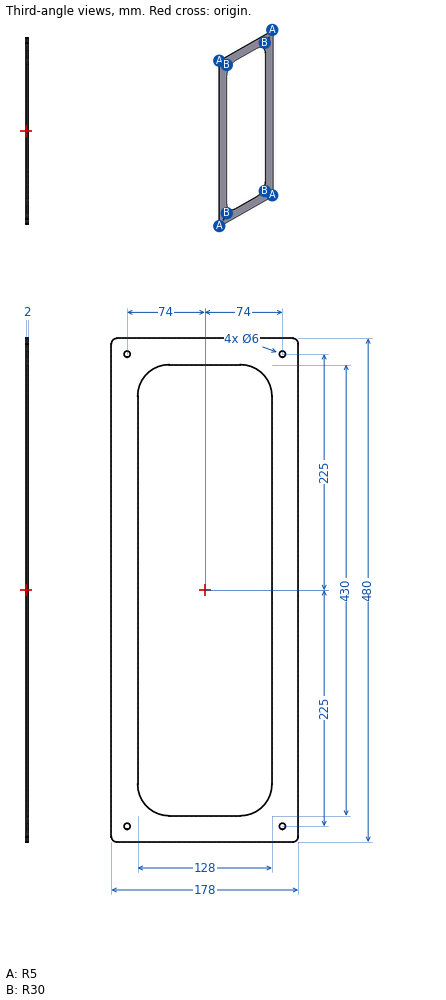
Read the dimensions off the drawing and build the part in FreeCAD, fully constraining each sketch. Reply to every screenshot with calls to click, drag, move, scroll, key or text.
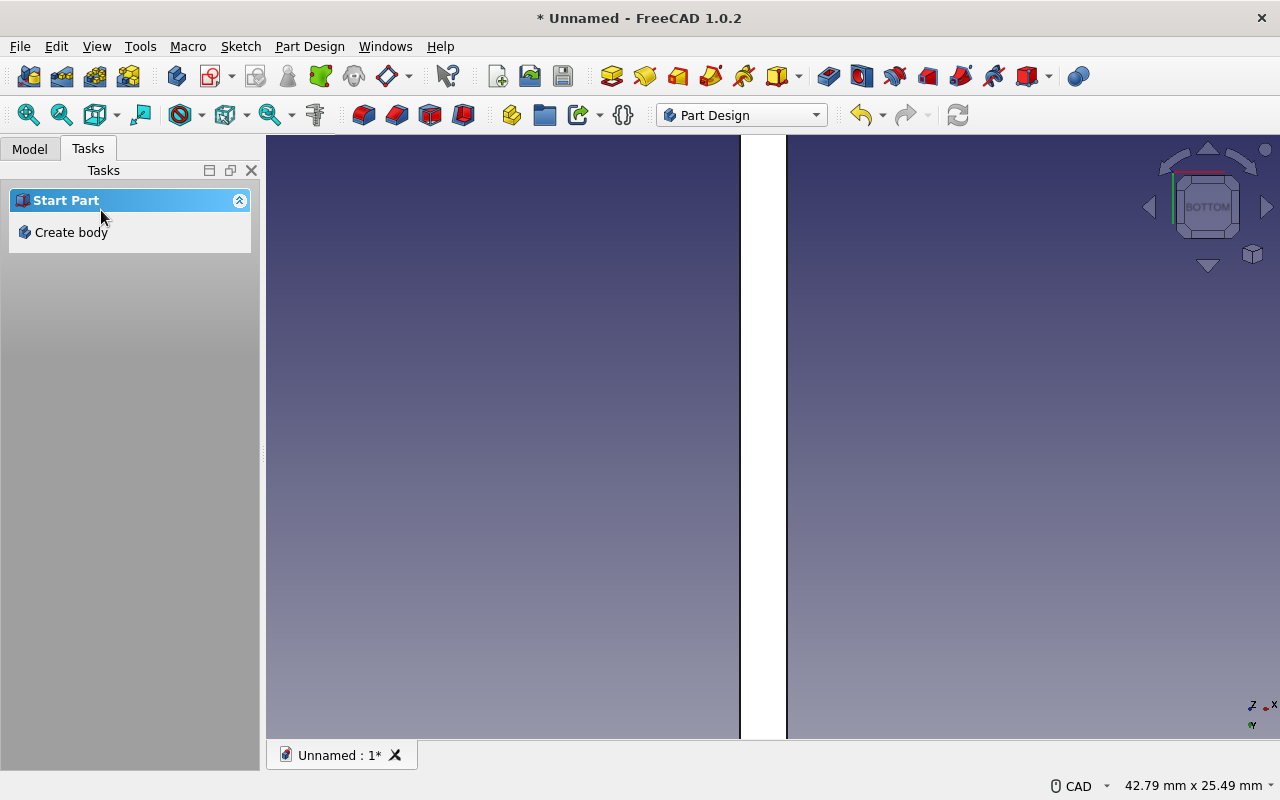
key(0)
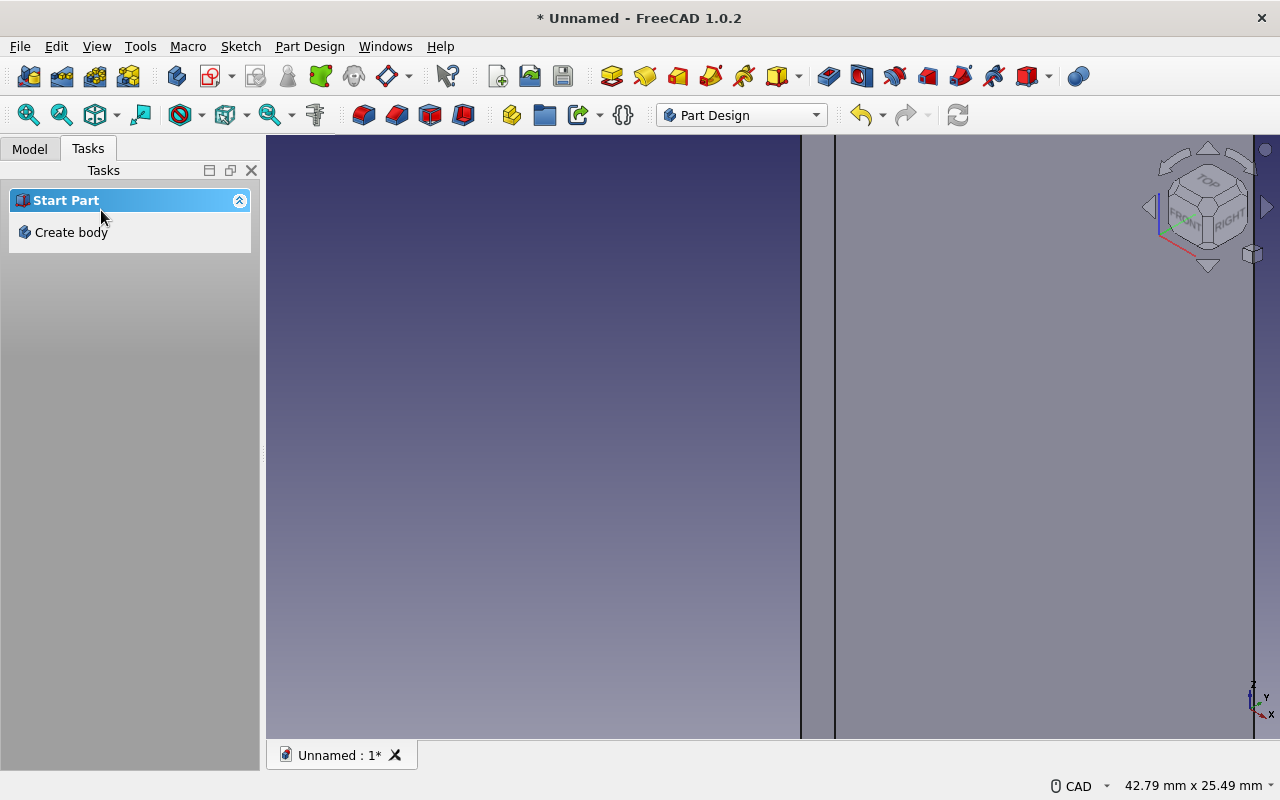
key(v)
key(f)